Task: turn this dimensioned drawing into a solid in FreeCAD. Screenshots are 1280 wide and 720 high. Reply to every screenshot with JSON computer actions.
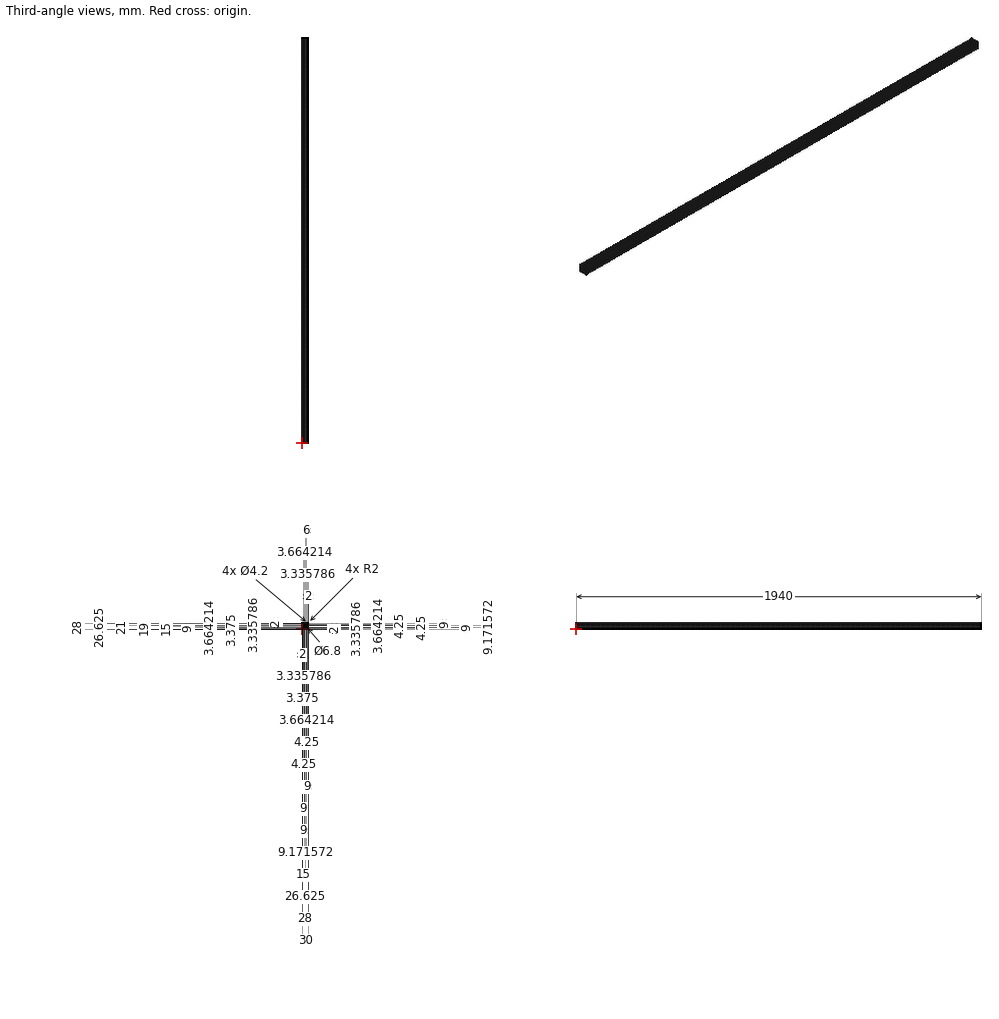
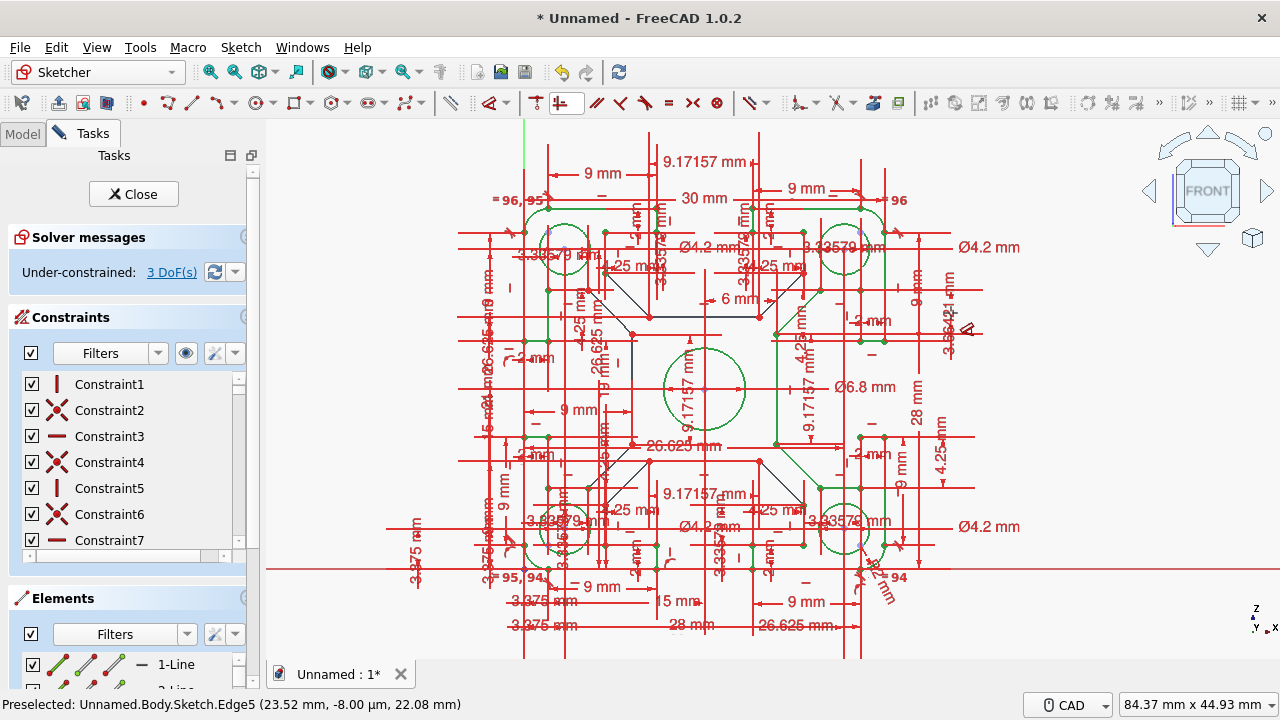
{"action": "left_click", "coordinate": [790, 492]}
{"action": "left_click", "coordinate": [792, 427]}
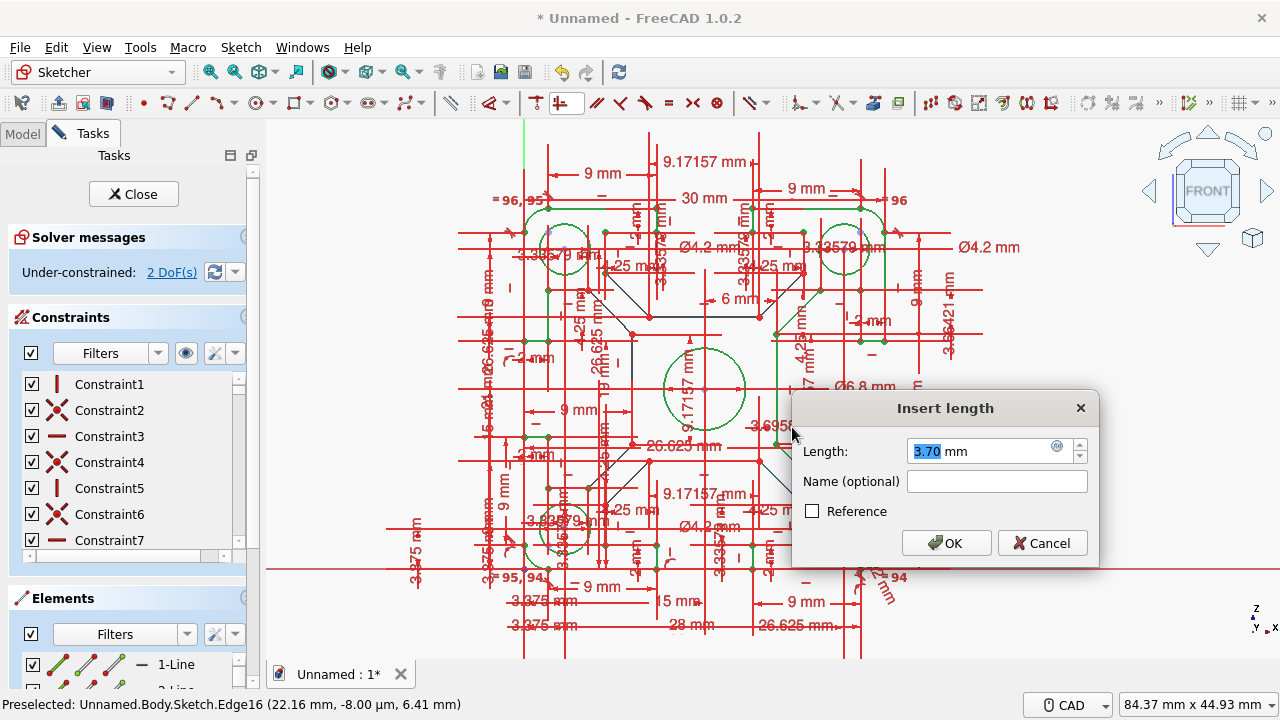
{"action": "type", "text": "3.664214"}
{"action": "key", "text": "Return"}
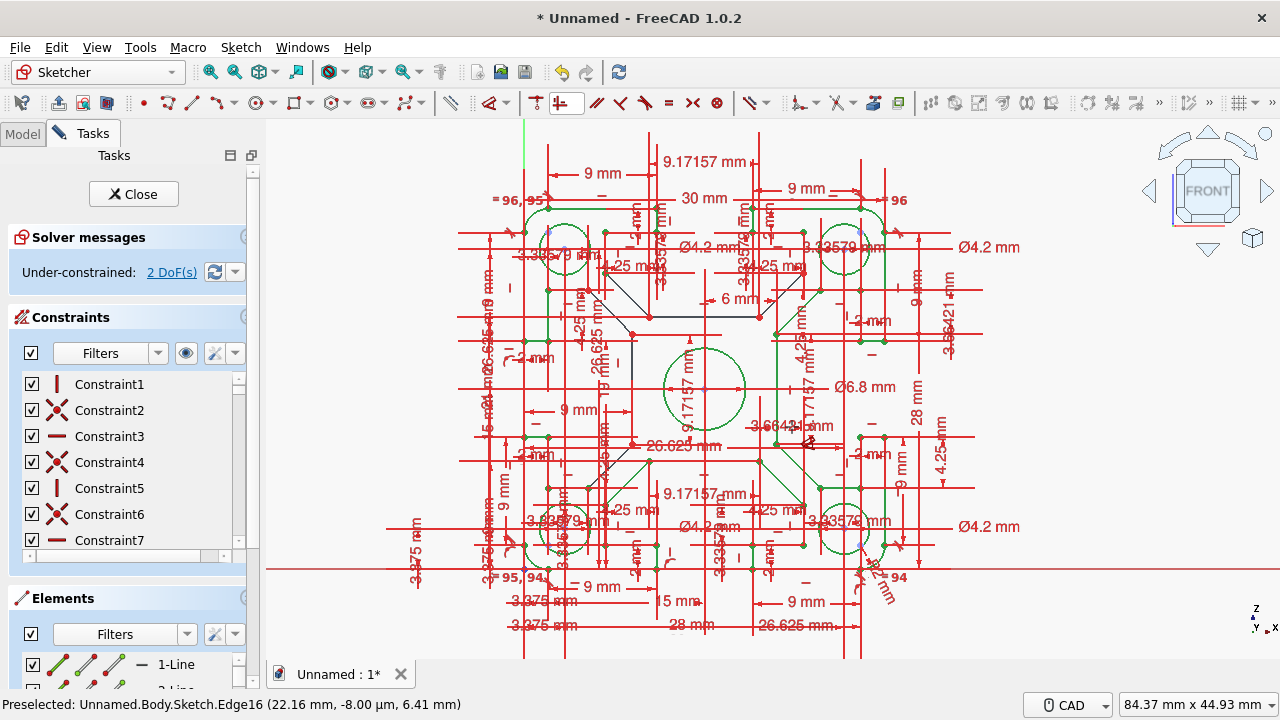
{"action": "left_click", "coordinate": [602, 475]}
{"action": "left_click", "coordinate": [458, 467]}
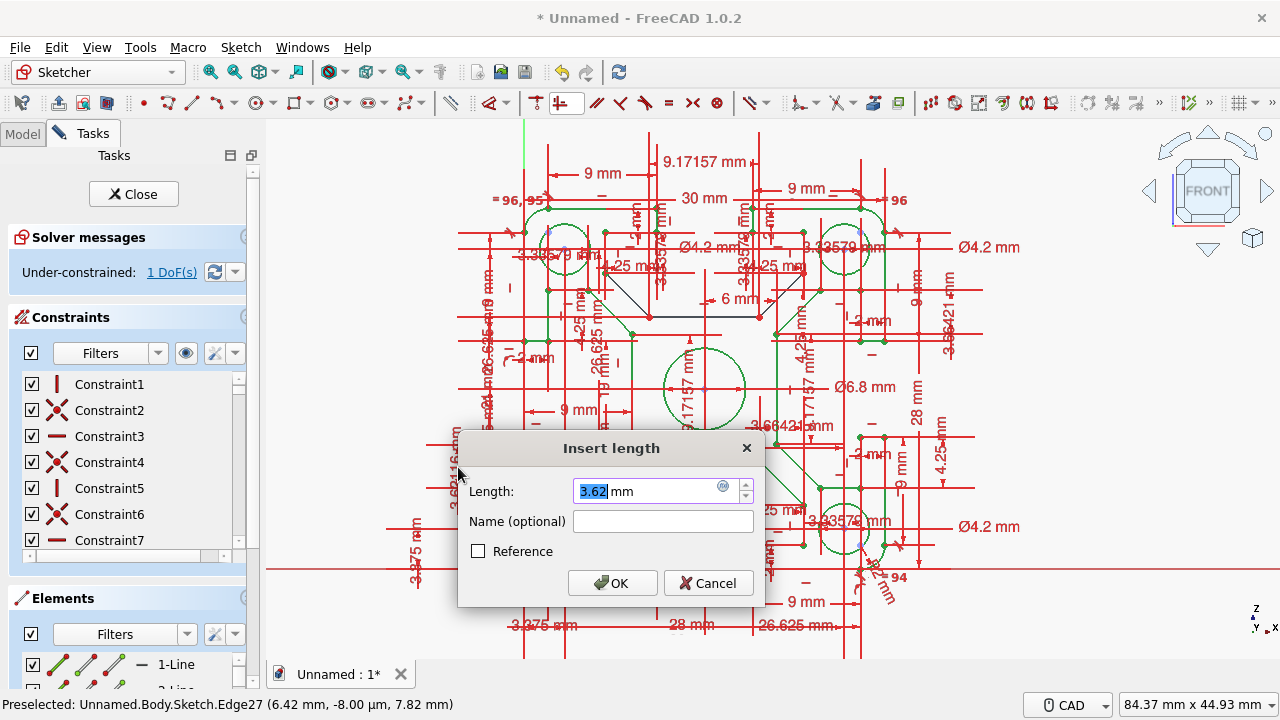
{"action": "type", "text": "3.664214"}
{"action": "key", "text": "Return"}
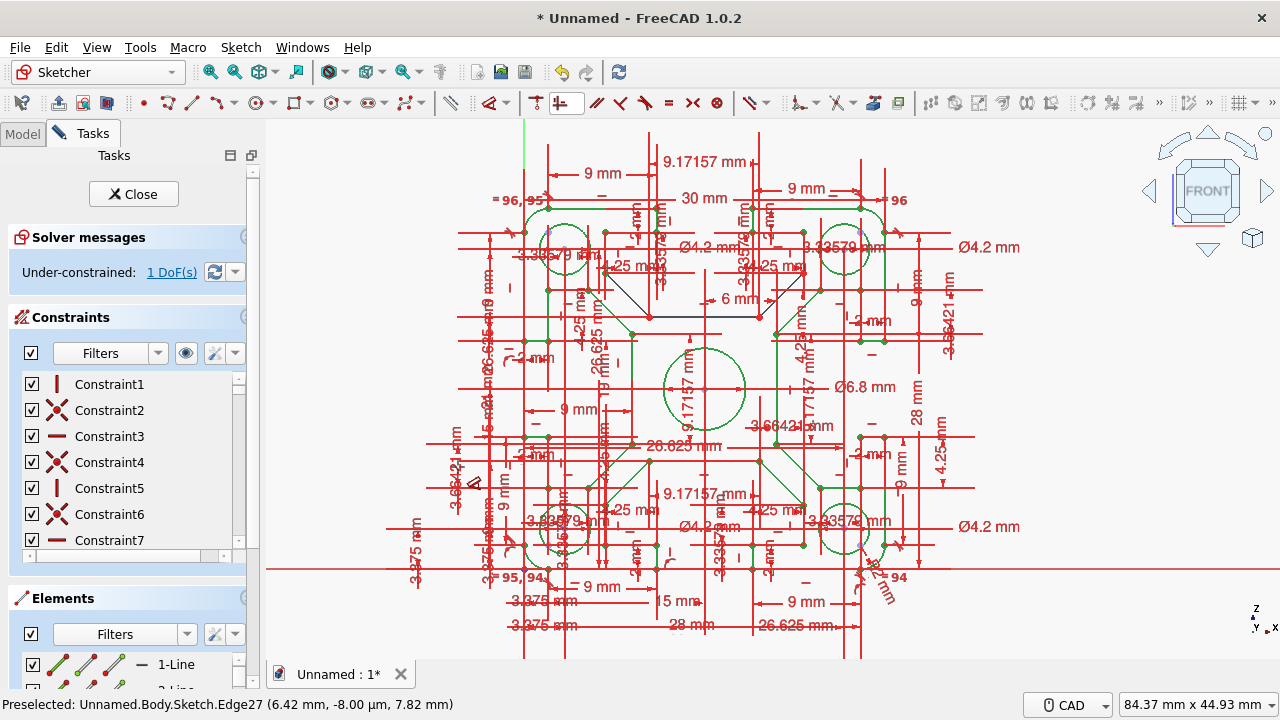
{"action": "left_click", "coordinate": [619, 286]}
{"action": "left_click", "coordinate": [617, 351]}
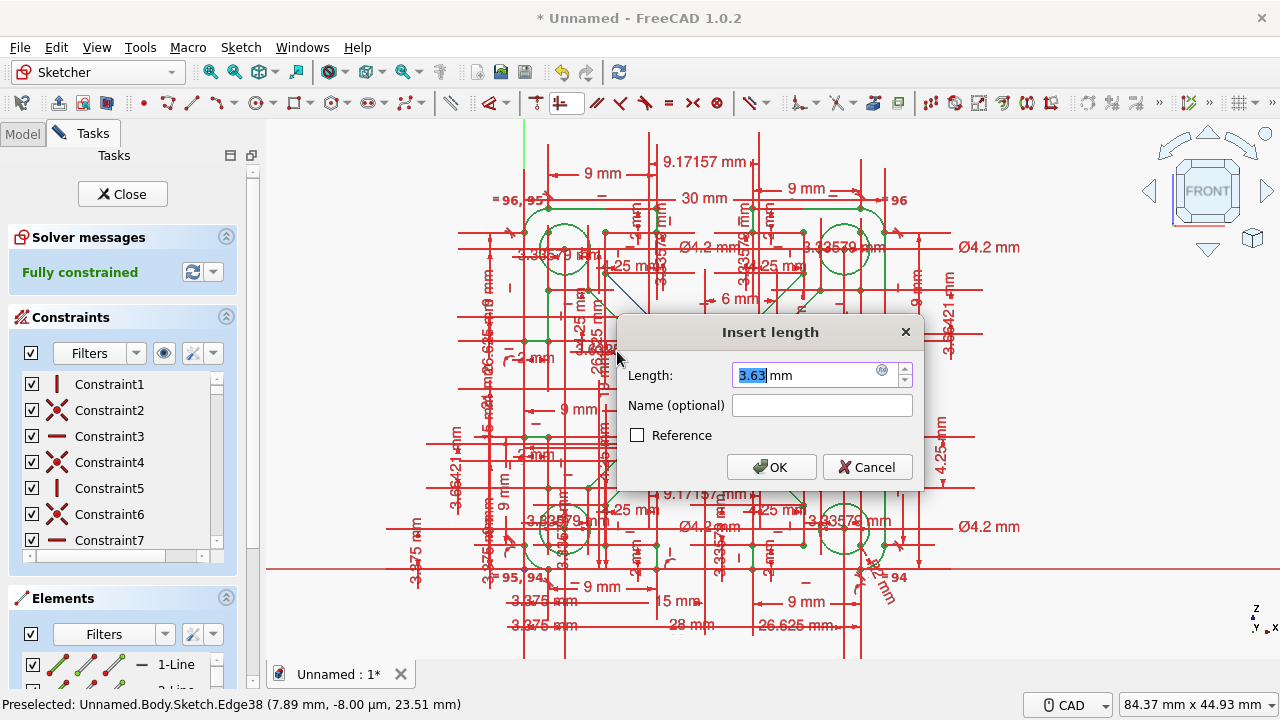
{"action": "type", "text": "3.664214"}
{"action": "key", "text": "Return"}
{"action": "key", "text": "Escape"}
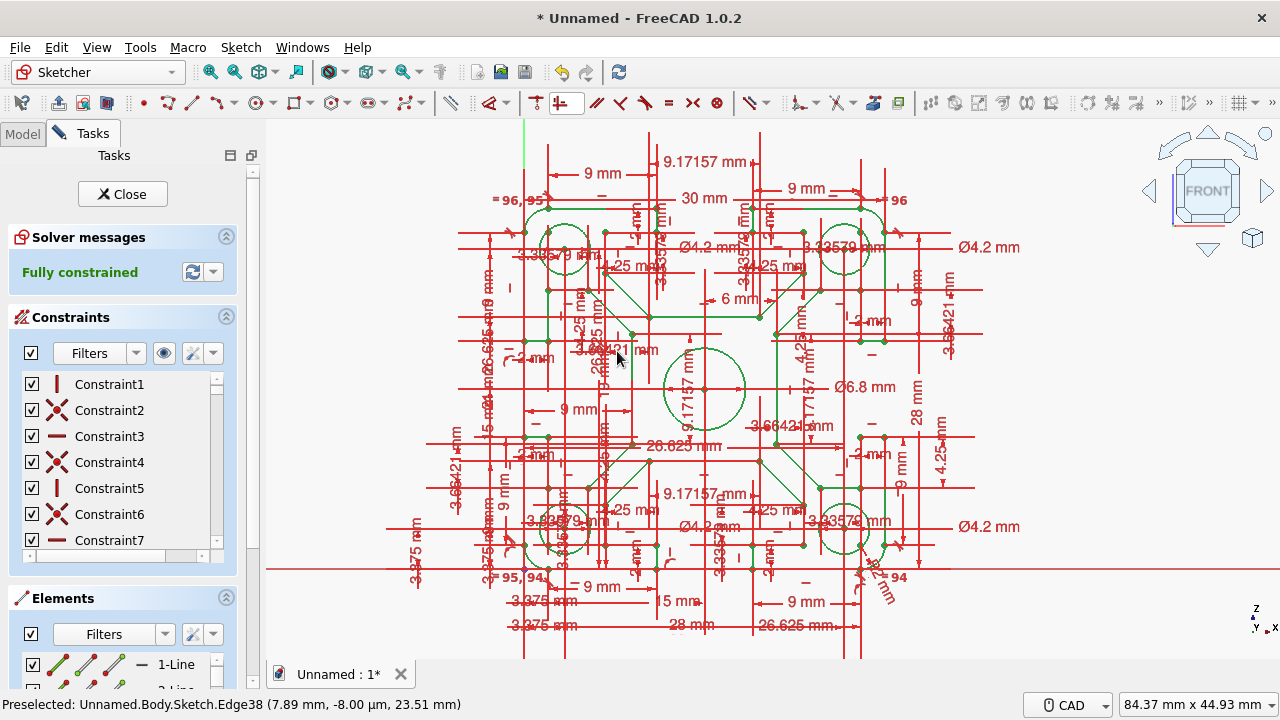
{"action": "left_click", "coordinate": [123, 194]}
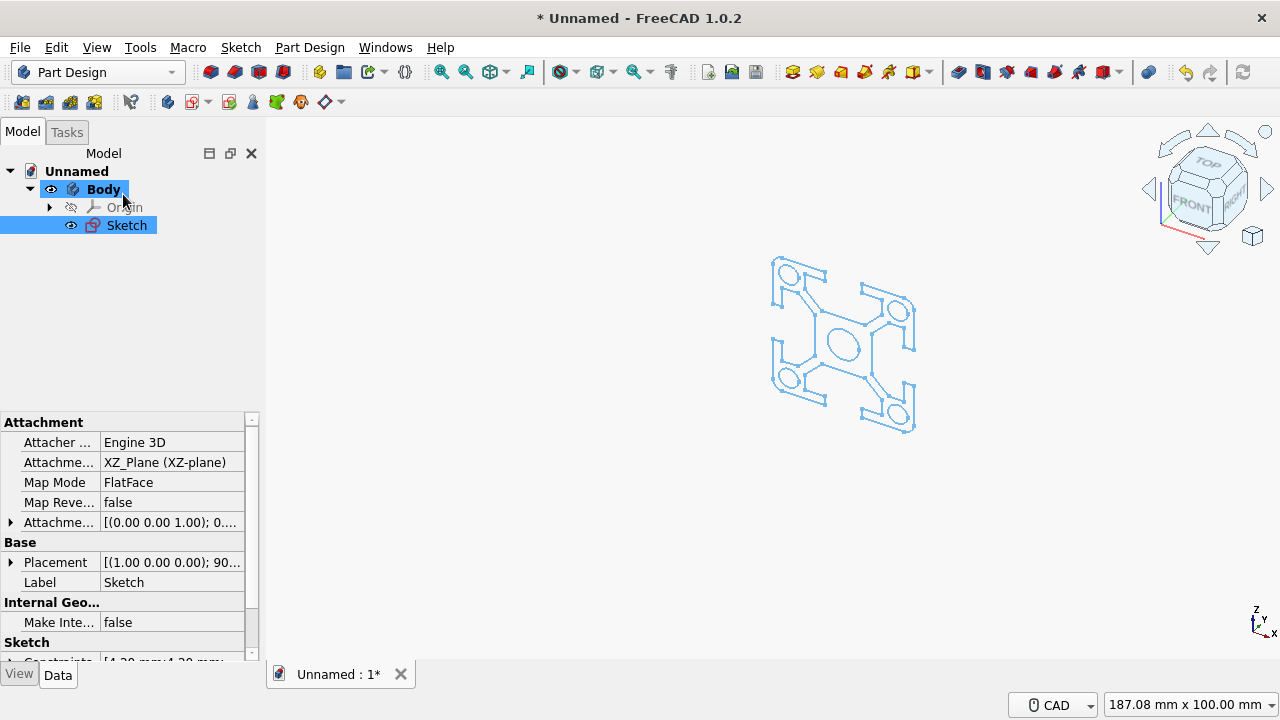
{"action": "left_click", "coordinate": [794, 72]}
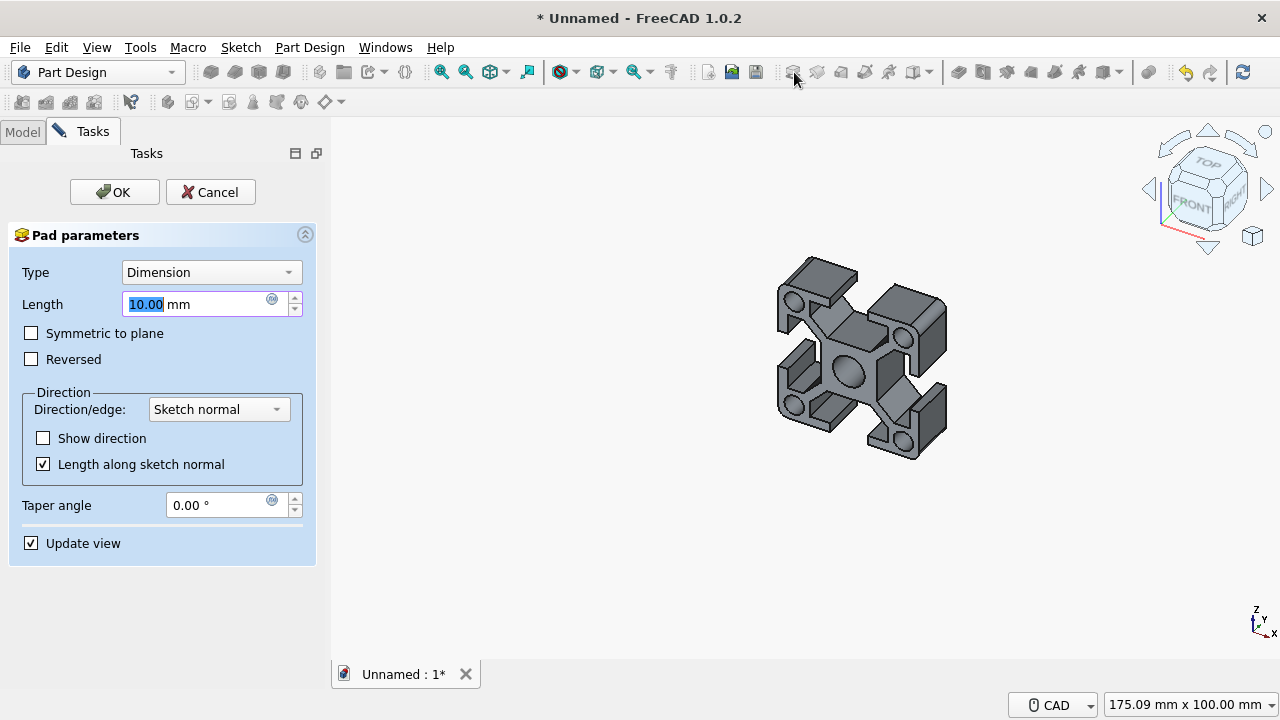
{"action": "type", "text": "1940"}
{"action": "key", "text": "Tab"}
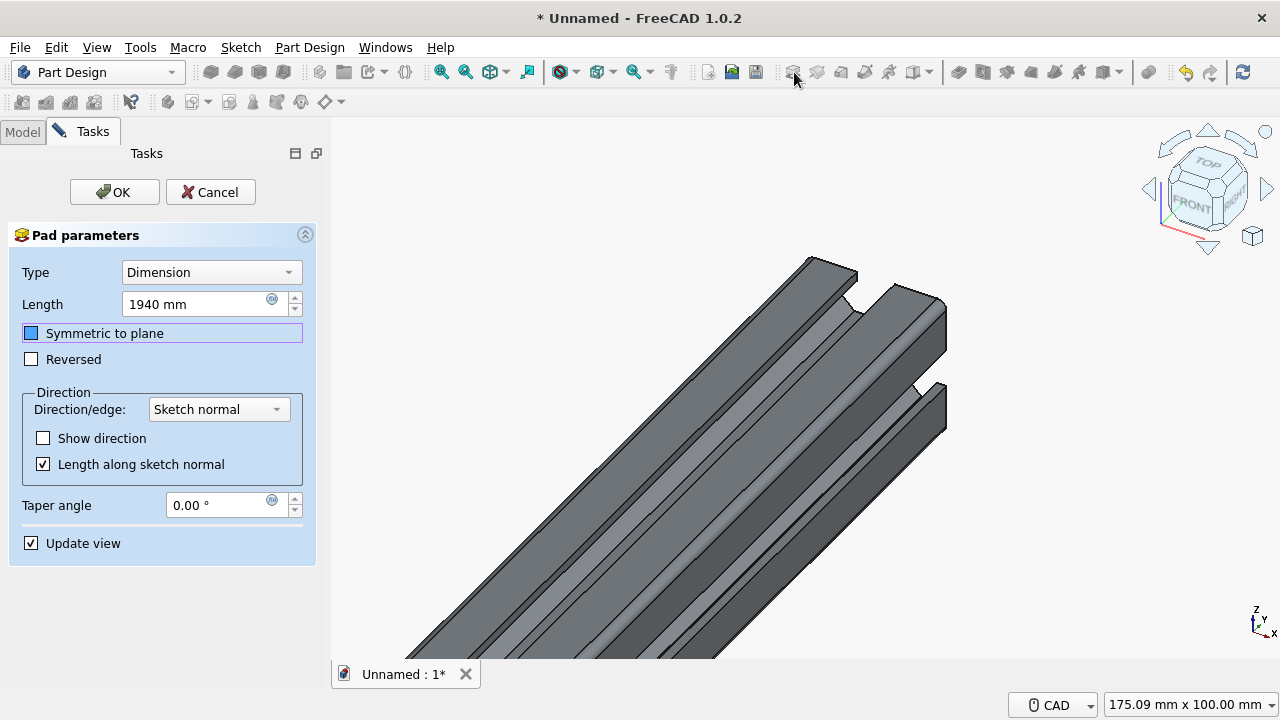
{"action": "left_click", "coordinate": [30, 359]}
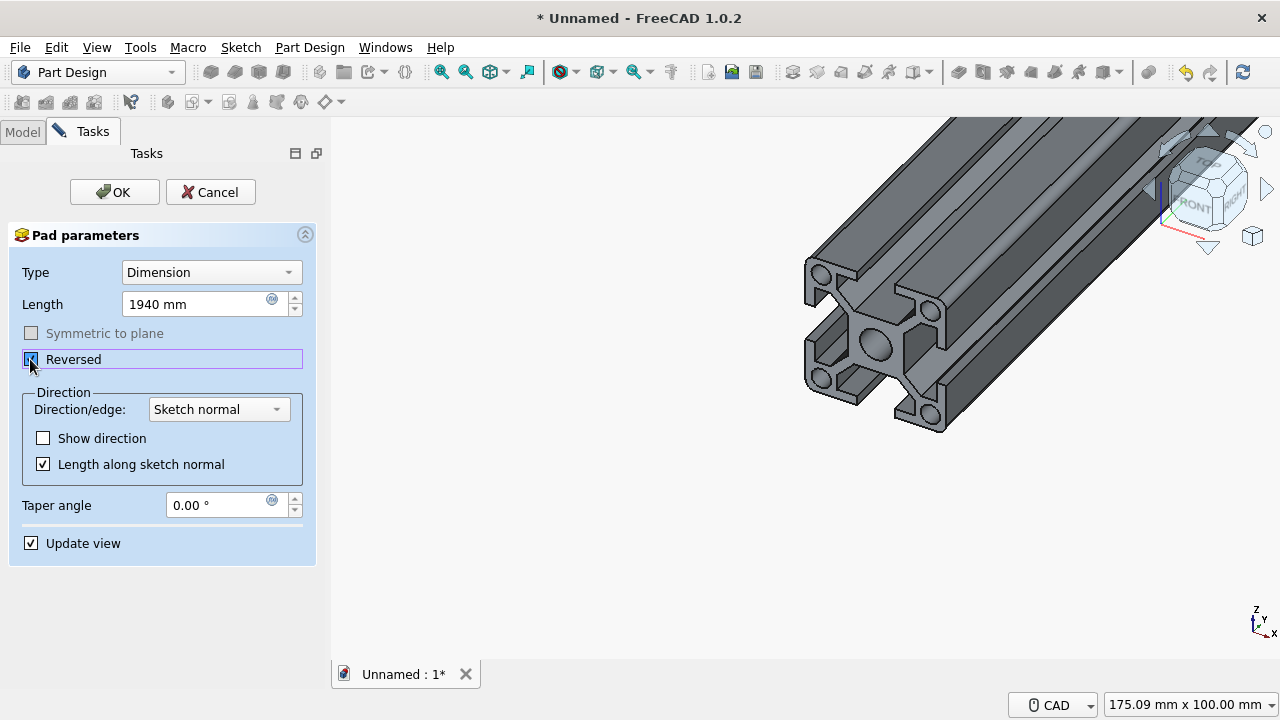
{"action": "left_click", "coordinate": [115, 192]}